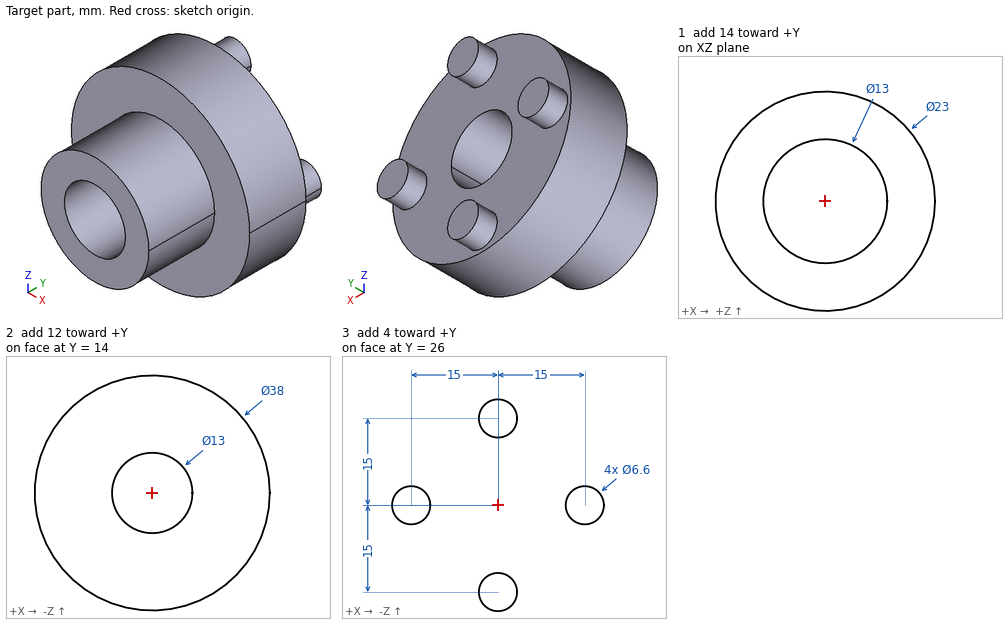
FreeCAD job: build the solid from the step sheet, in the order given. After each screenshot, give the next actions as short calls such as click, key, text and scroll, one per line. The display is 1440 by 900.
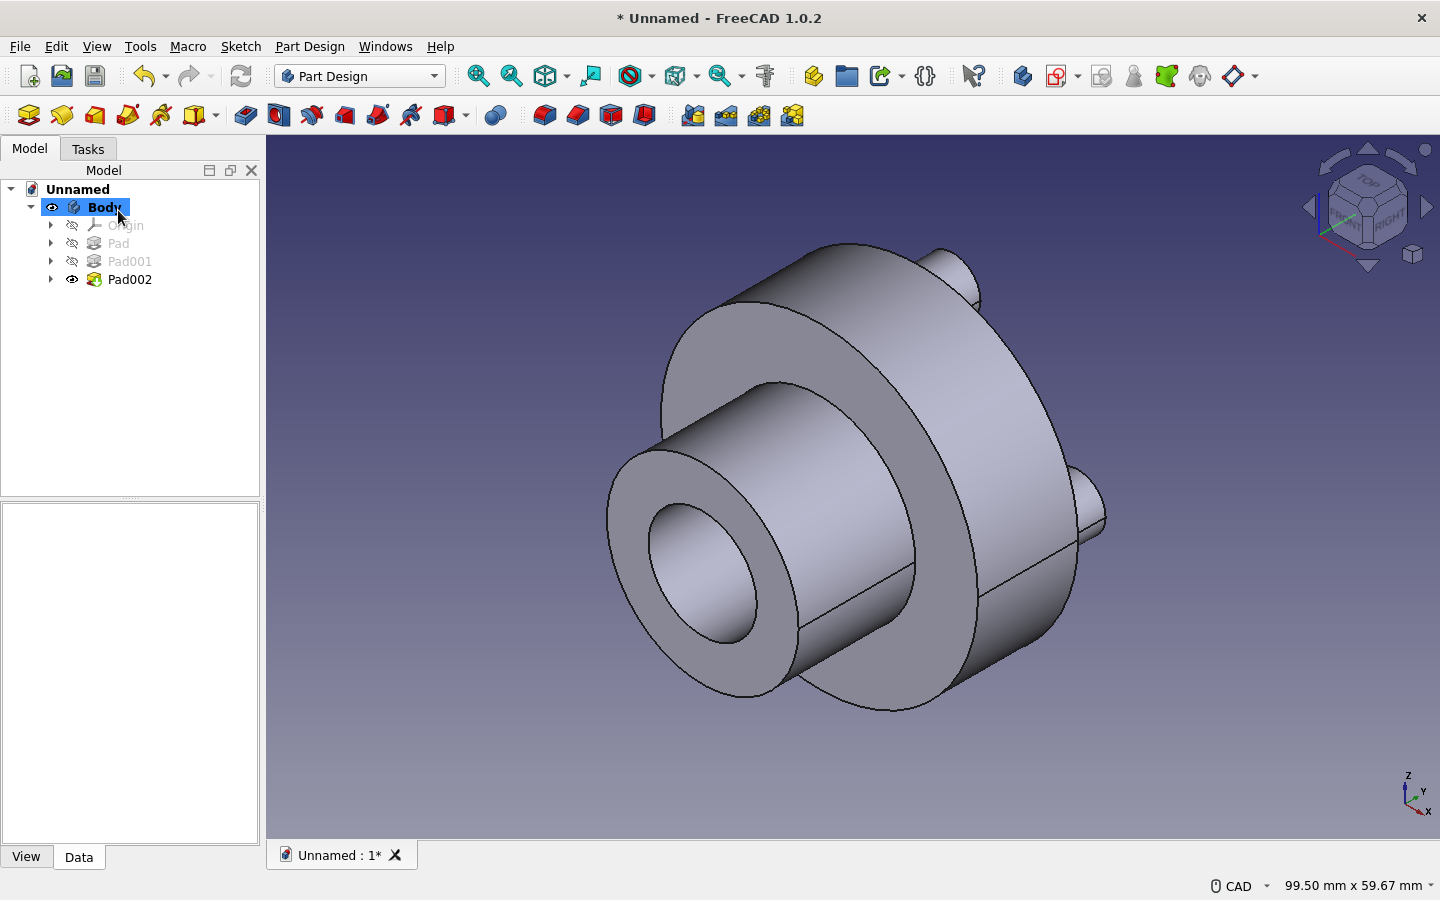
key(v)
key(f)